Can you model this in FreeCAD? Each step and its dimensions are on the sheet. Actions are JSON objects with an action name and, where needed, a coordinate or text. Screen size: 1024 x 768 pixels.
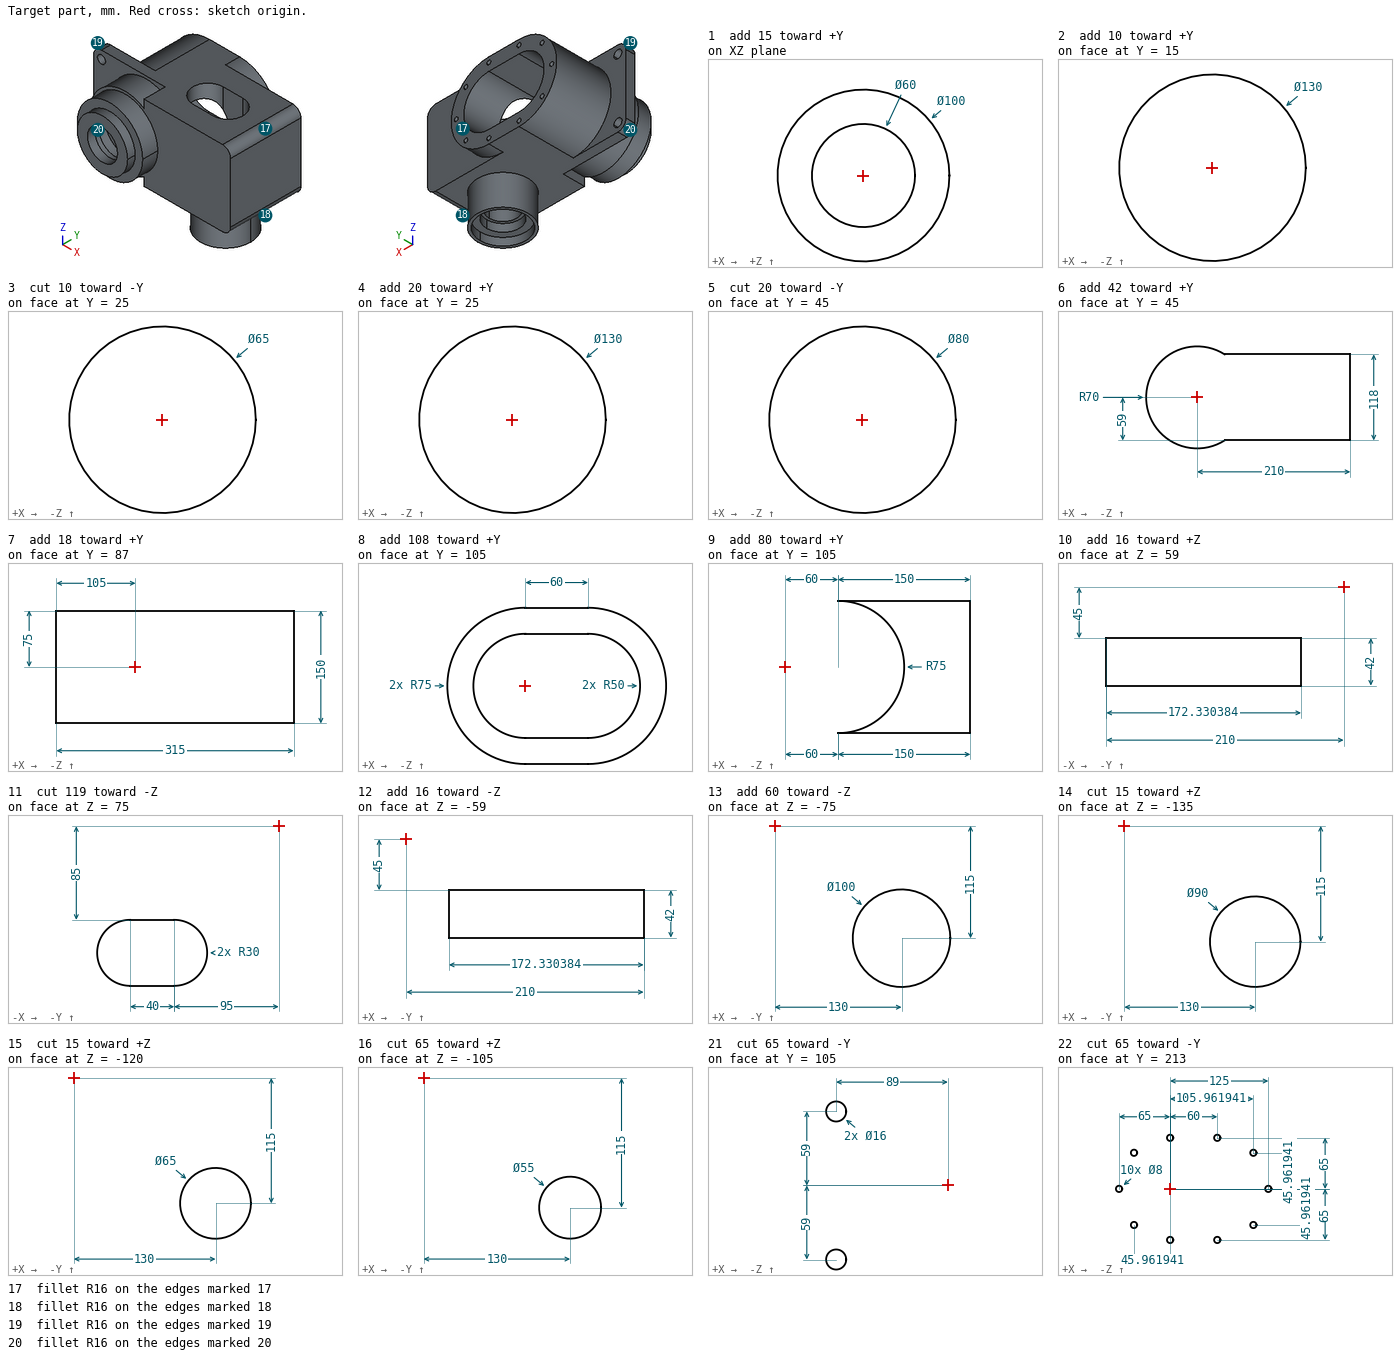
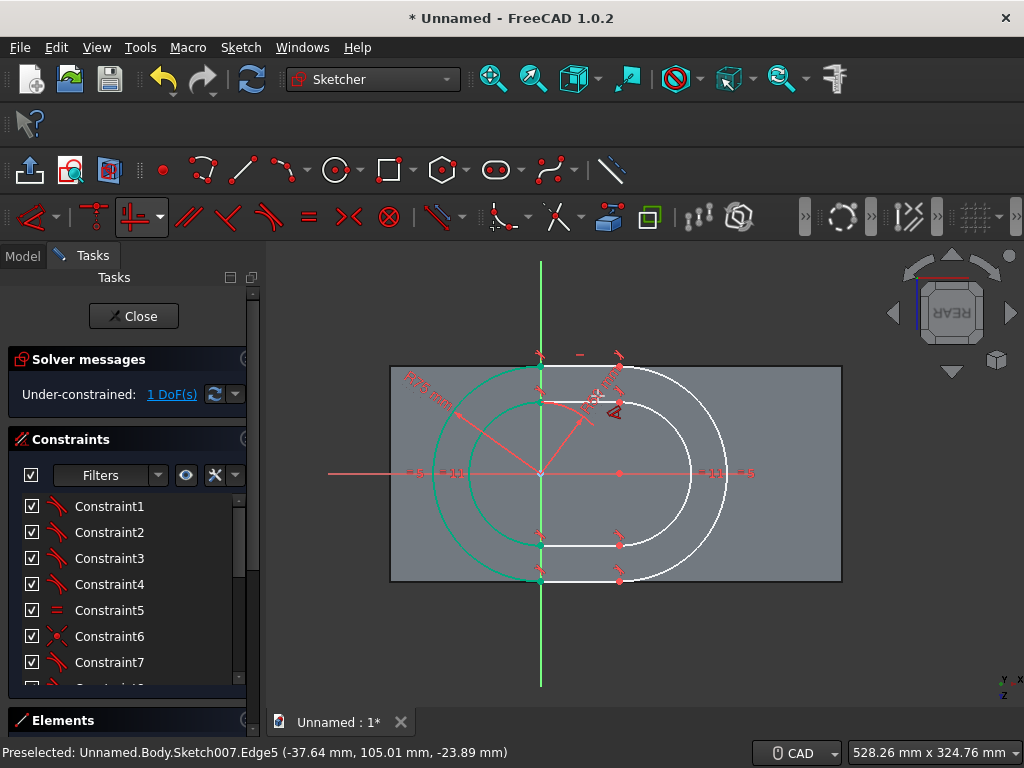
{"action": "left_click", "coordinate": [564, 366]}
{"action": "left_click", "coordinate": [580, 332]}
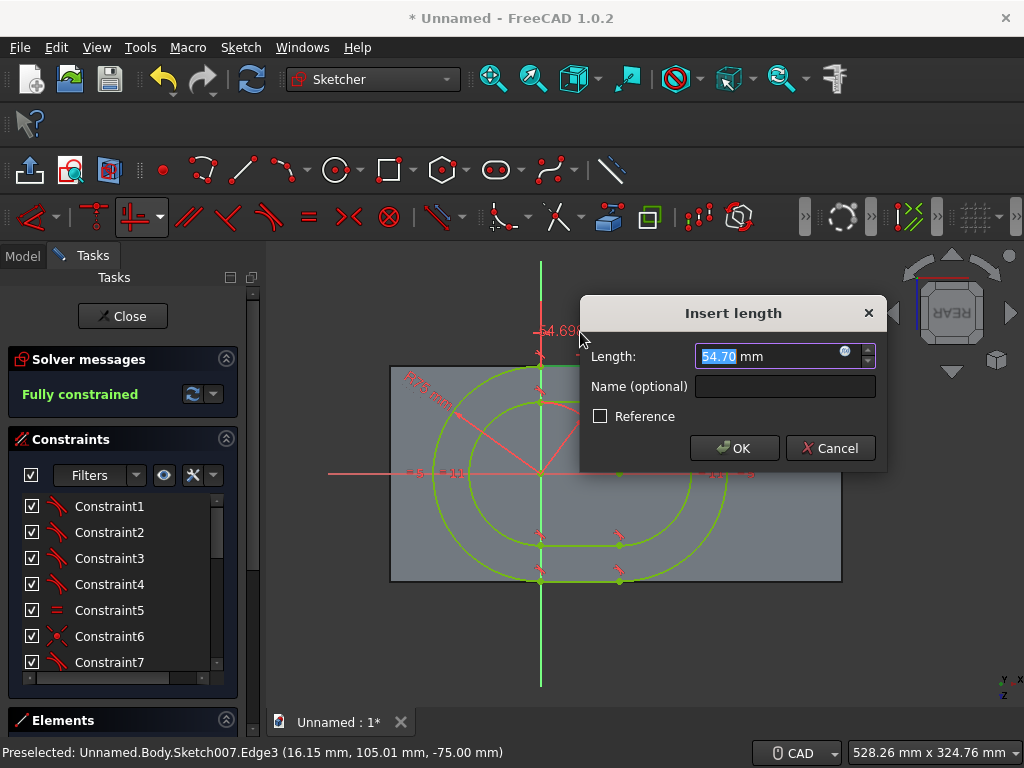
{"action": "type", "text": "60"}
{"action": "key", "text": "Return"}
{"action": "key", "text": "Escape"}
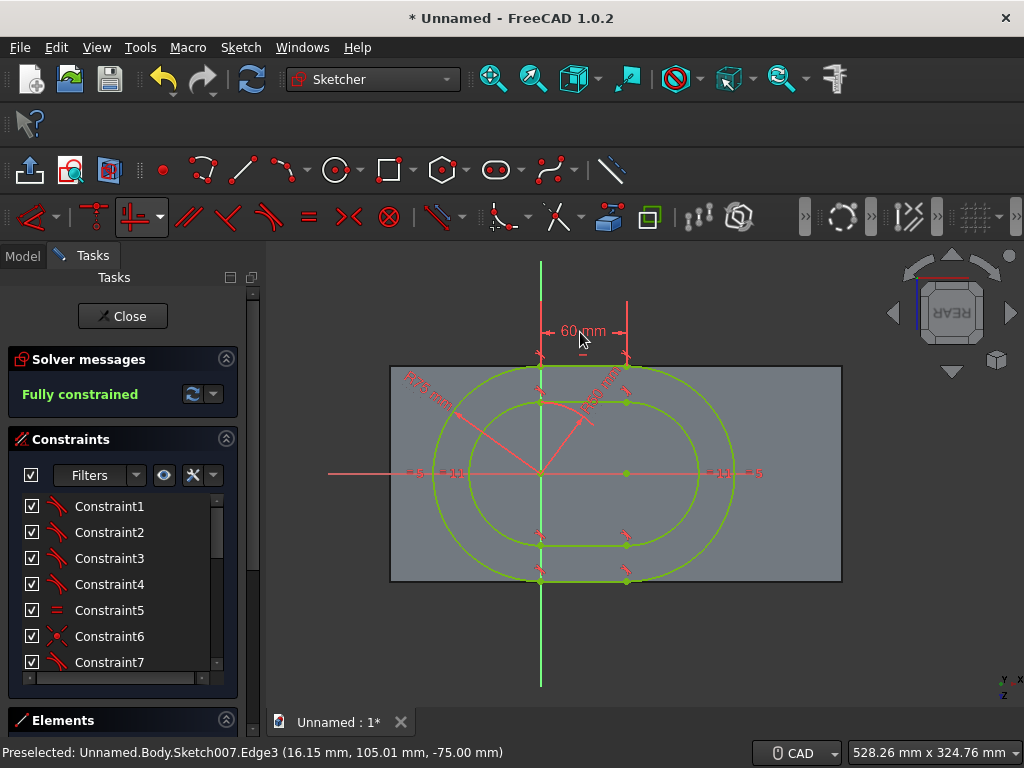
{"action": "left_click", "coordinate": [123, 316]}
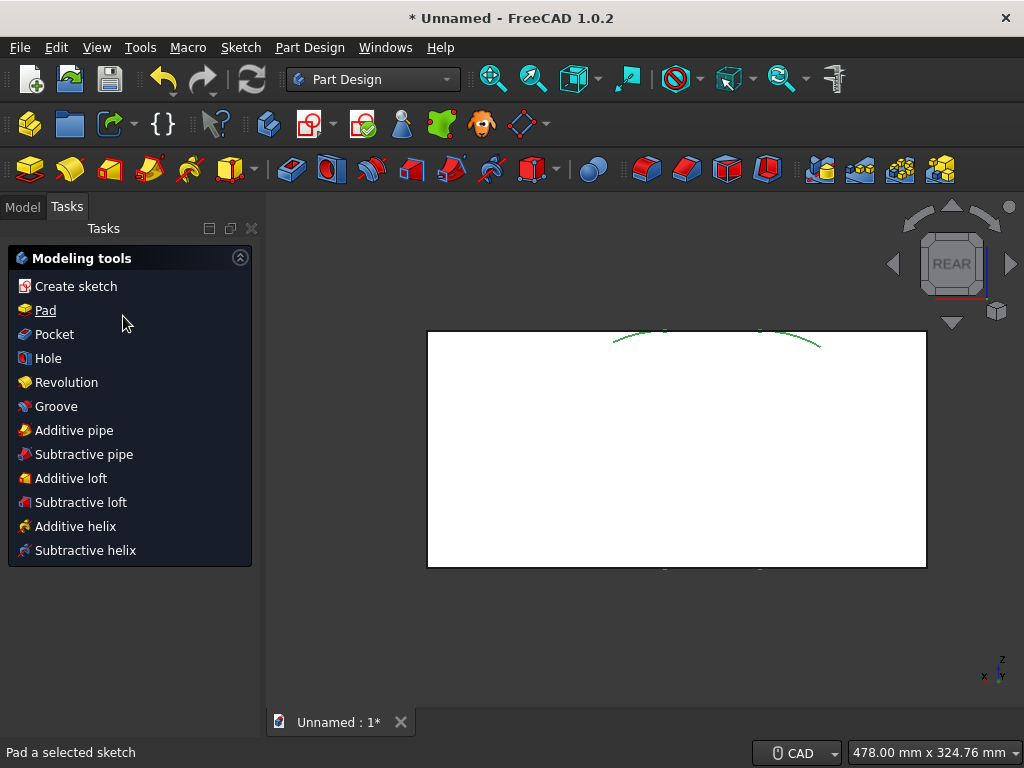
{"action": "left_click", "coordinate": [30, 170]}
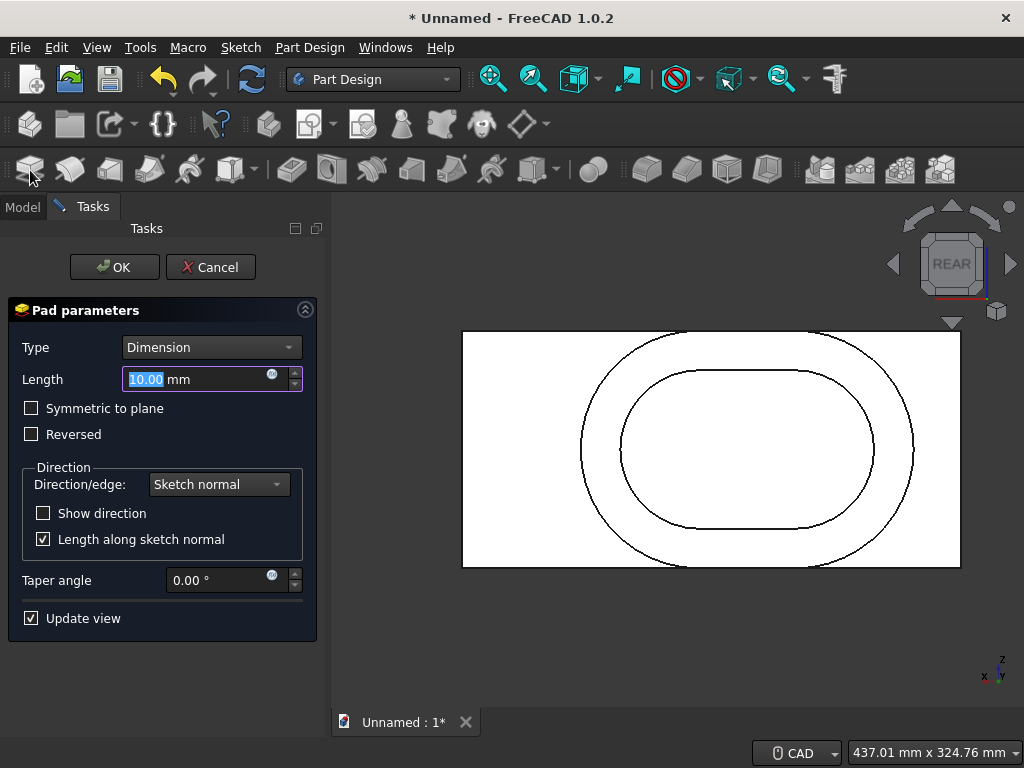
{"action": "type", "text": "108"}
{"action": "key", "text": "Tab"}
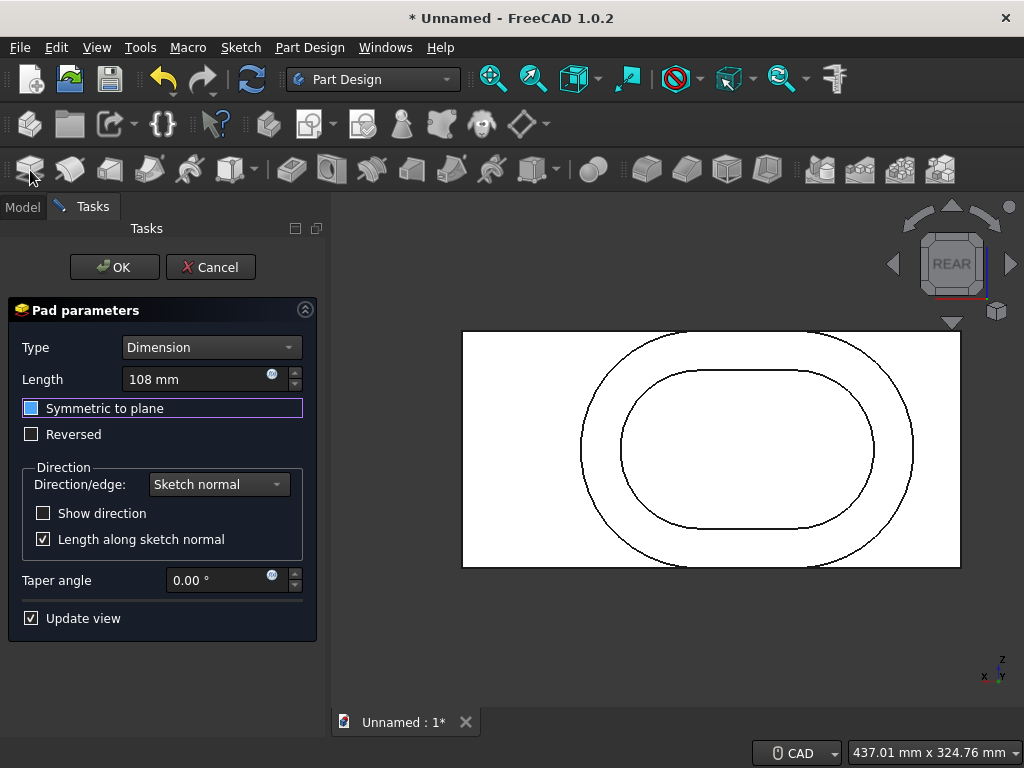
{"action": "left_click", "coordinate": [115, 267]}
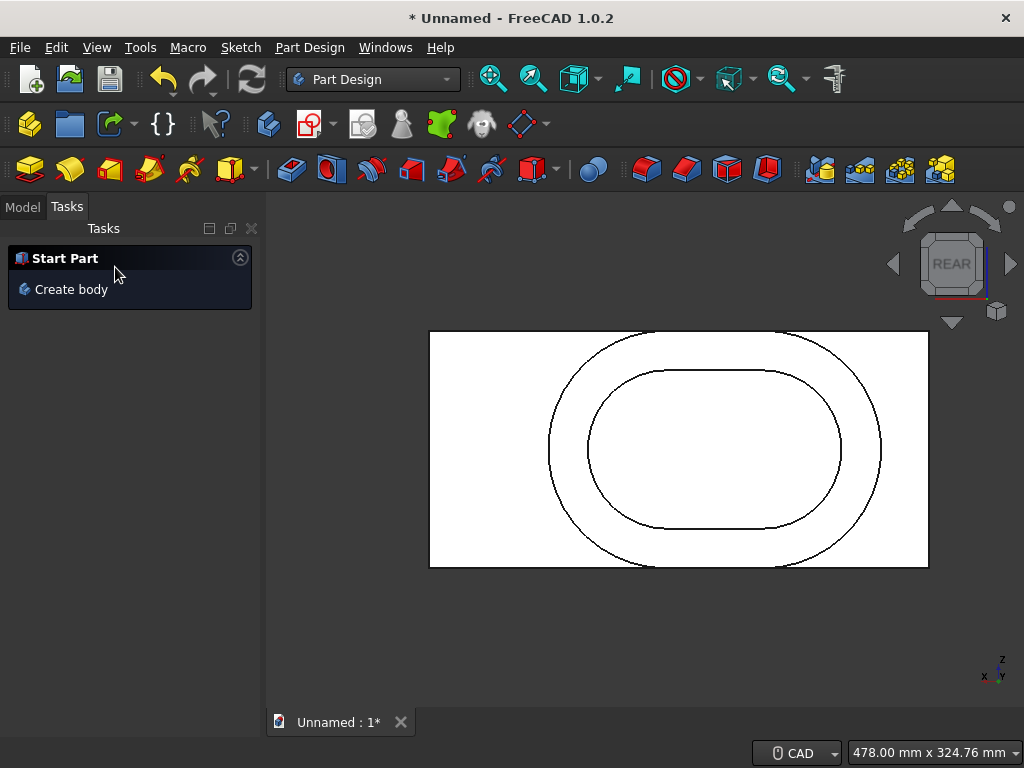
{"action": "left_click", "coordinate": [678, 448]}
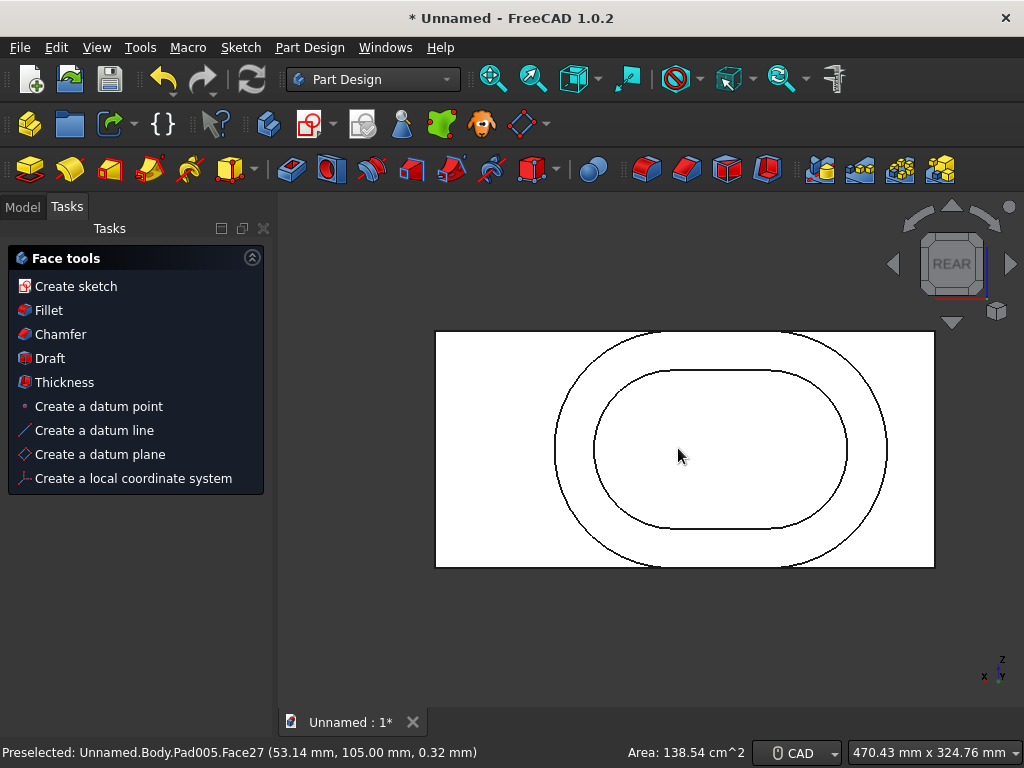
{"action": "left_click", "coordinate": [310, 124]}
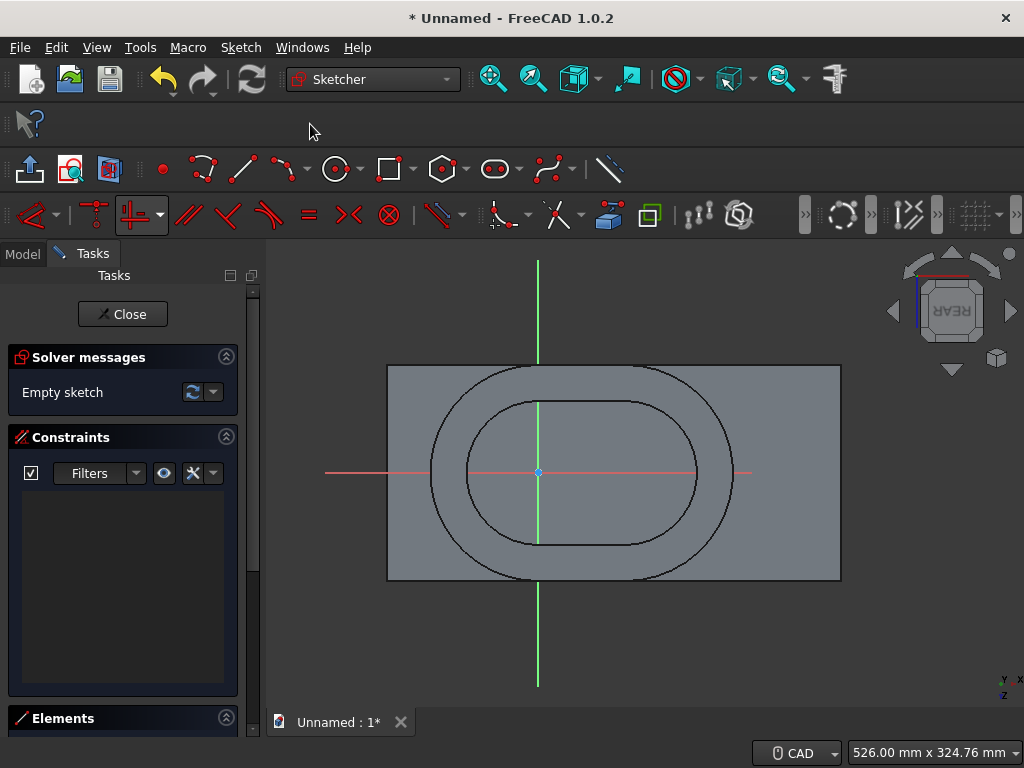
{"action": "scroll", "coordinate": [294, 473], "scroll_direction": "down", "scroll_amount": 1}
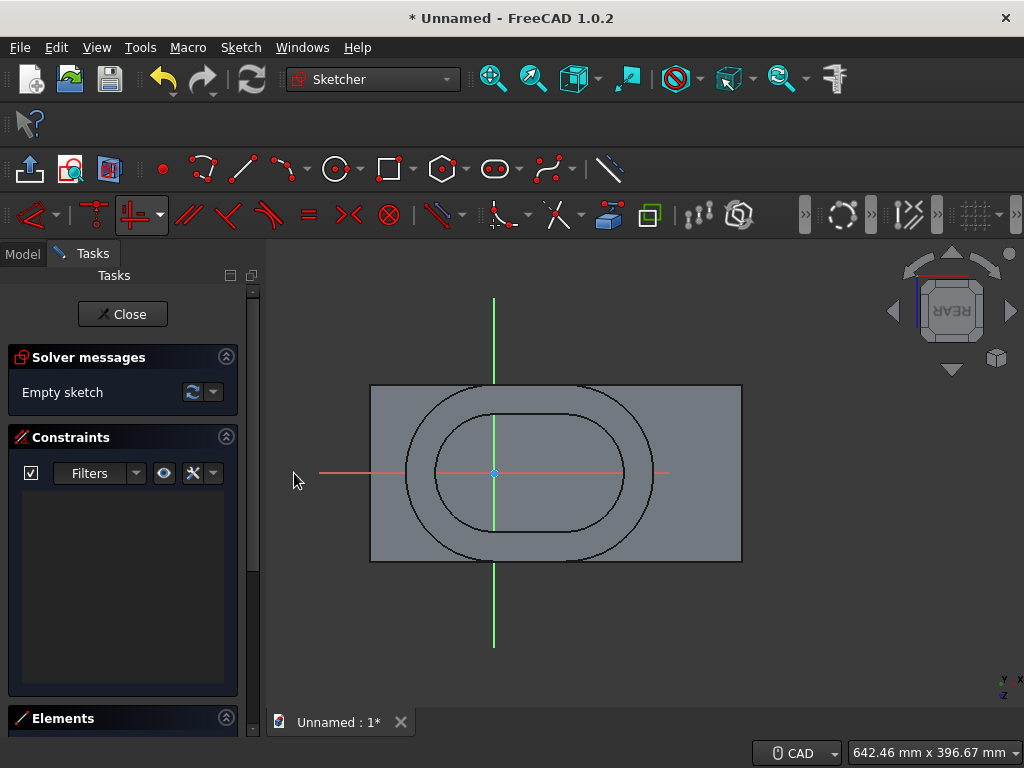
{"action": "scroll", "coordinate": [702, 473], "scroll_direction": "up", "scroll_amount": 2}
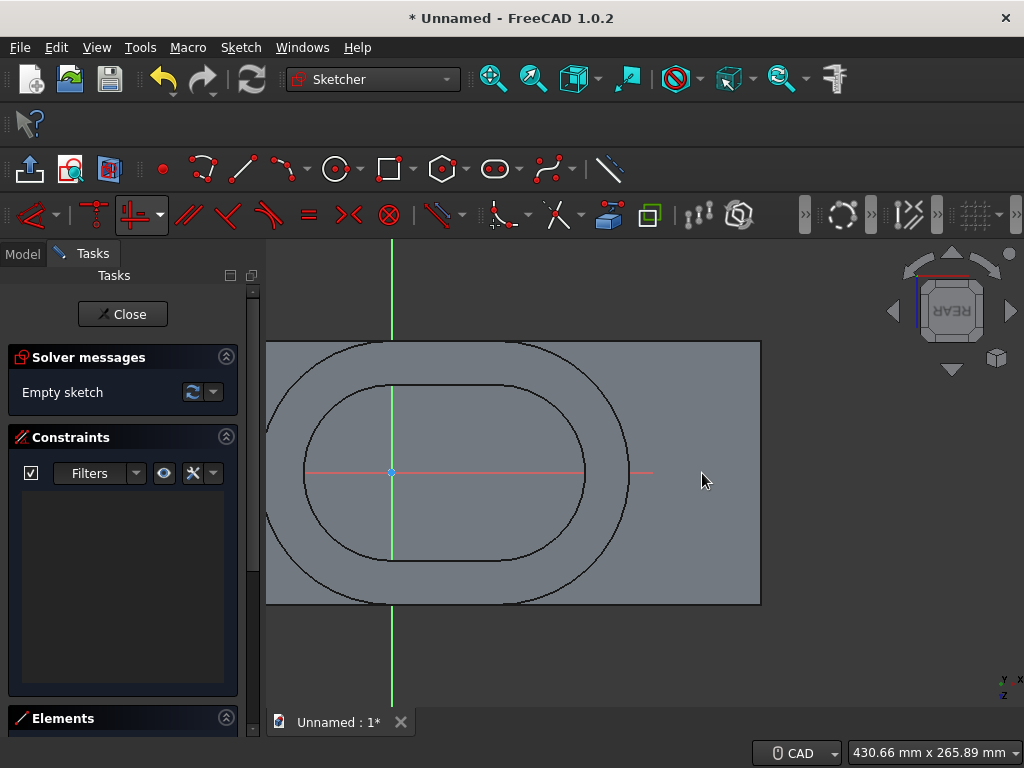
{"action": "left_click", "coordinate": [204, 170]}